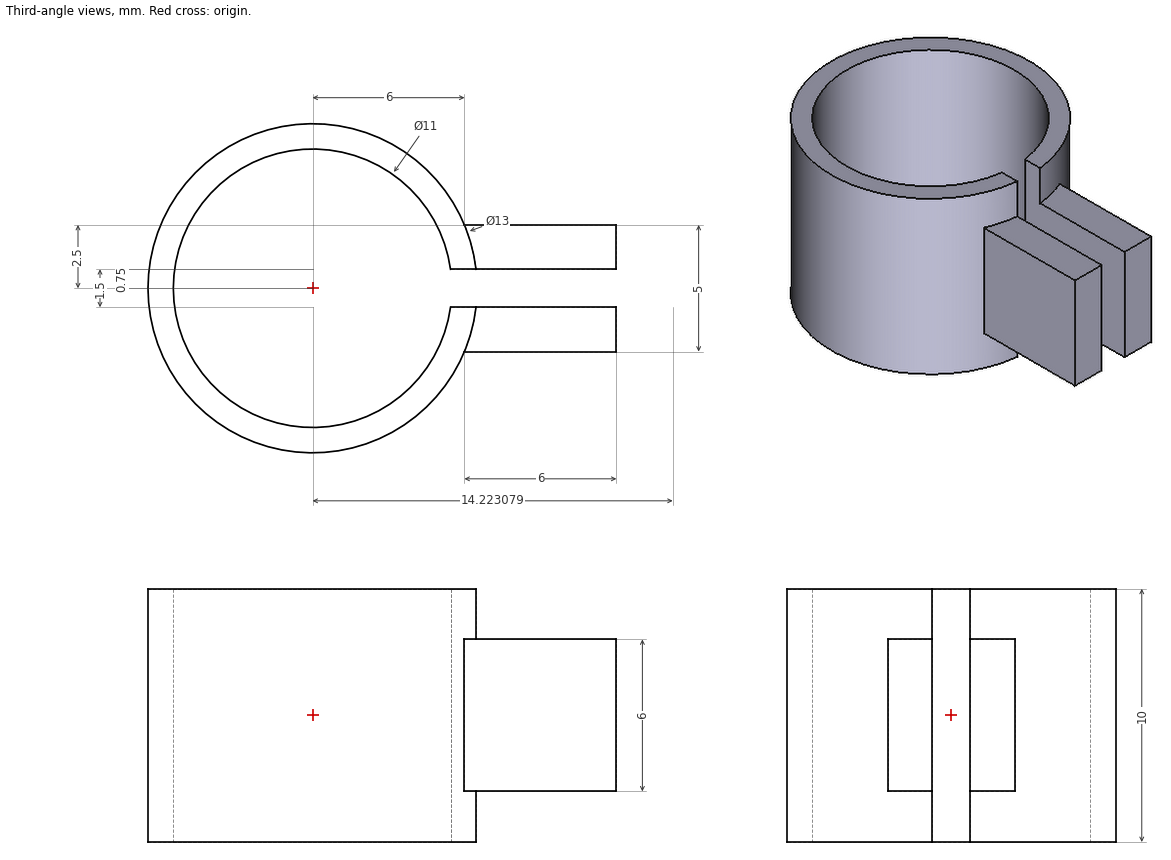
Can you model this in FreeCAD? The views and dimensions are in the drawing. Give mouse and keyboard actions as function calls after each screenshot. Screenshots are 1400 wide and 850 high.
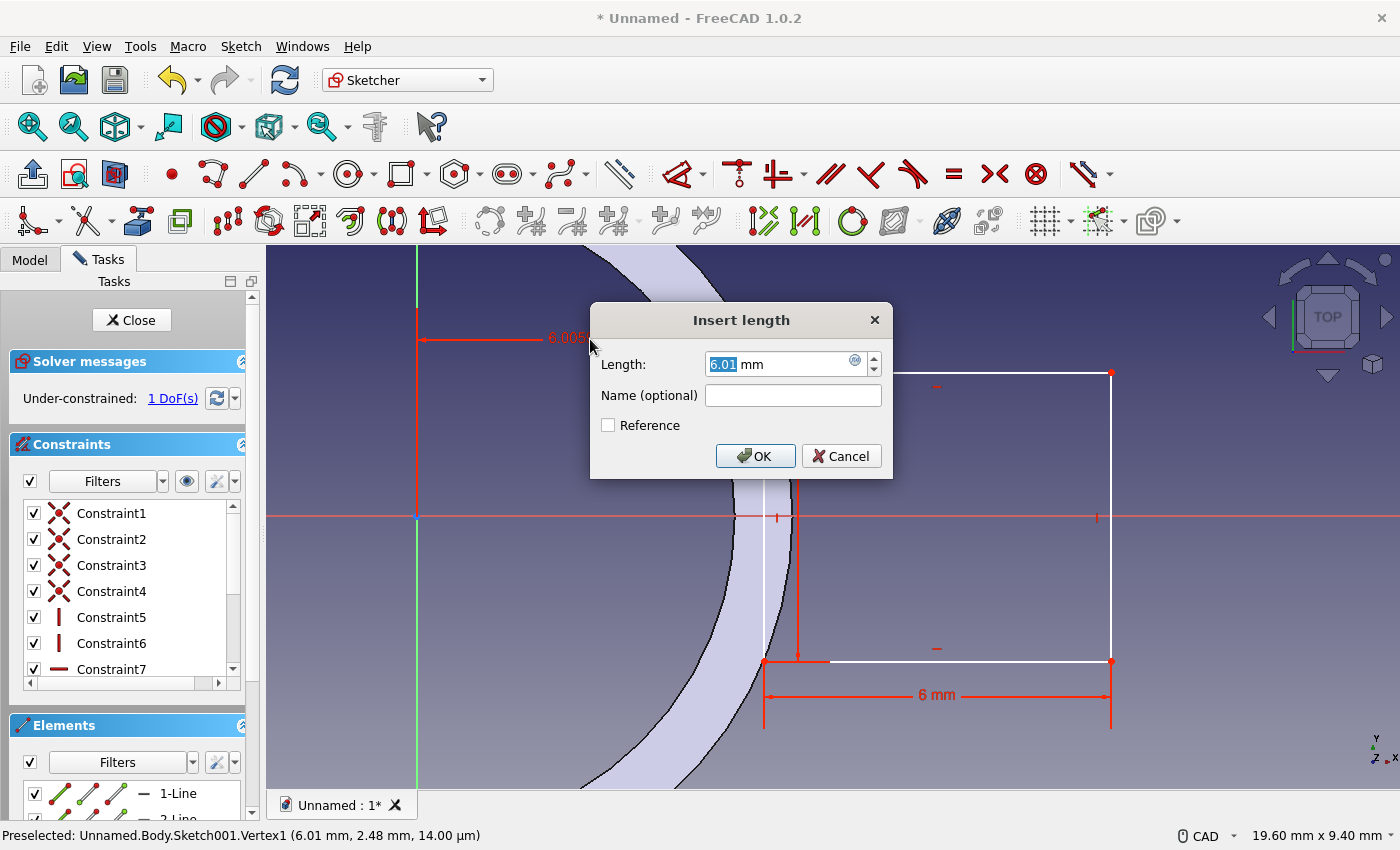
text(6)
key(Return)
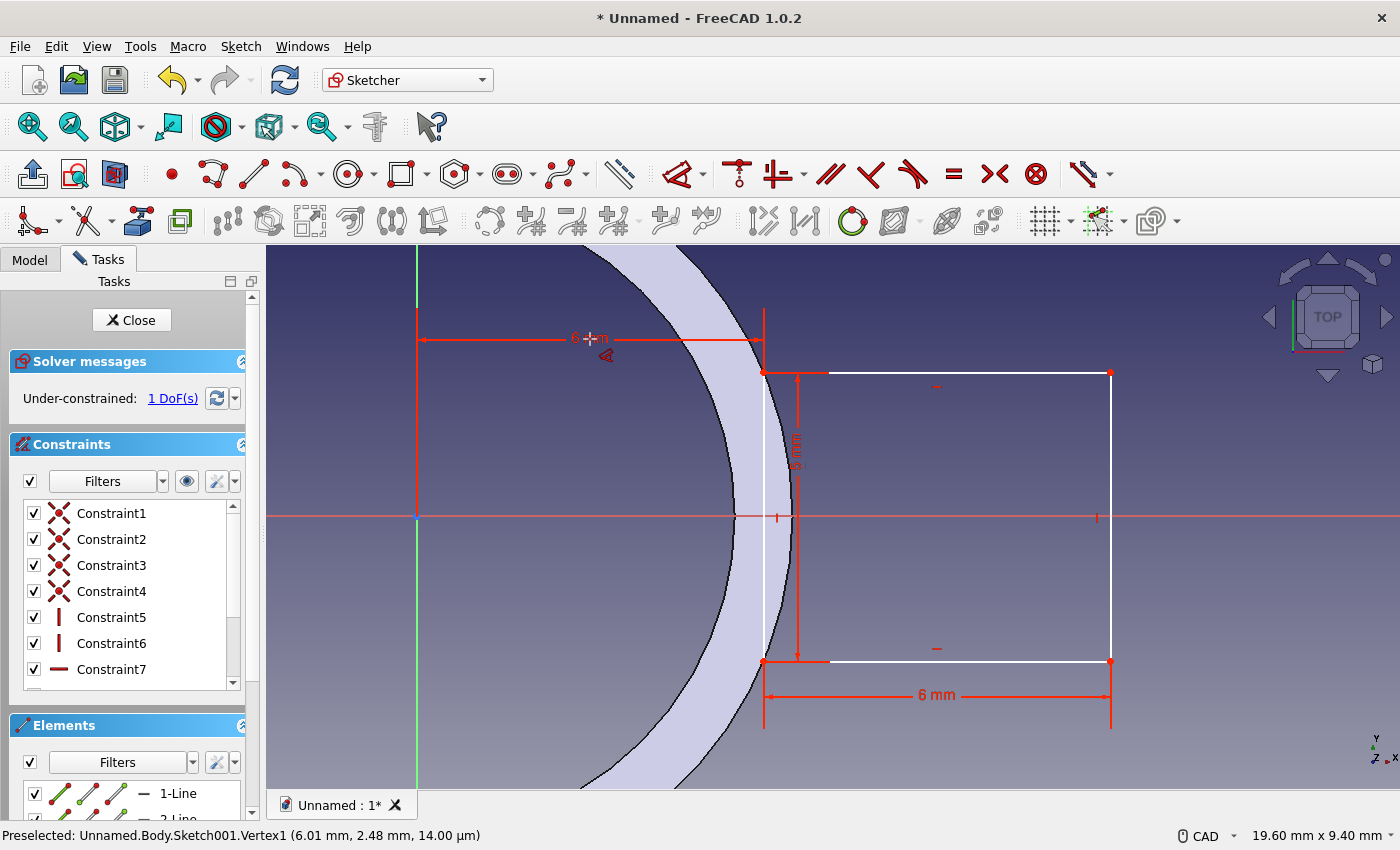
click(764, 373)
click(383, 445)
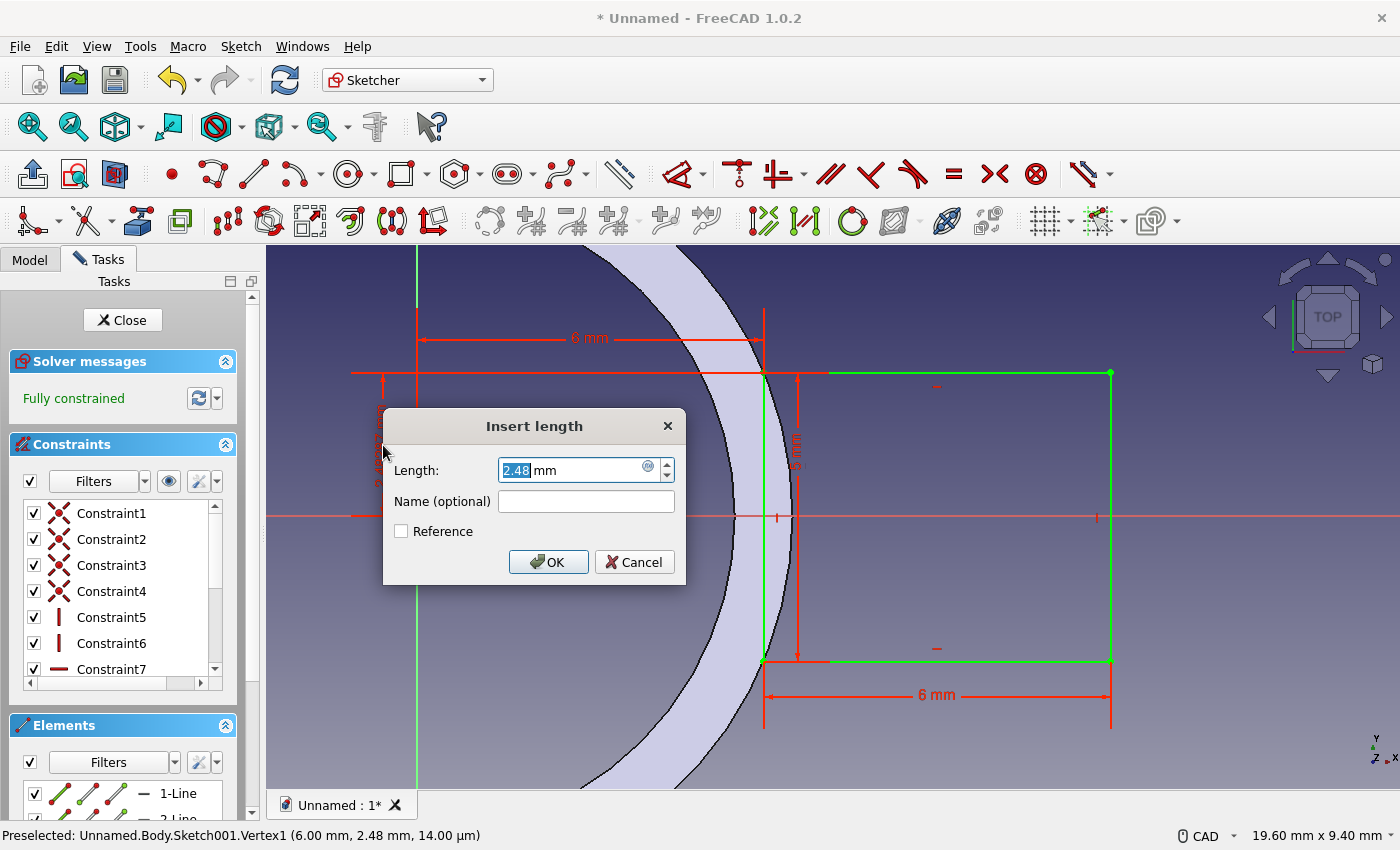
text(2.5)
key(Return)
key(Escape)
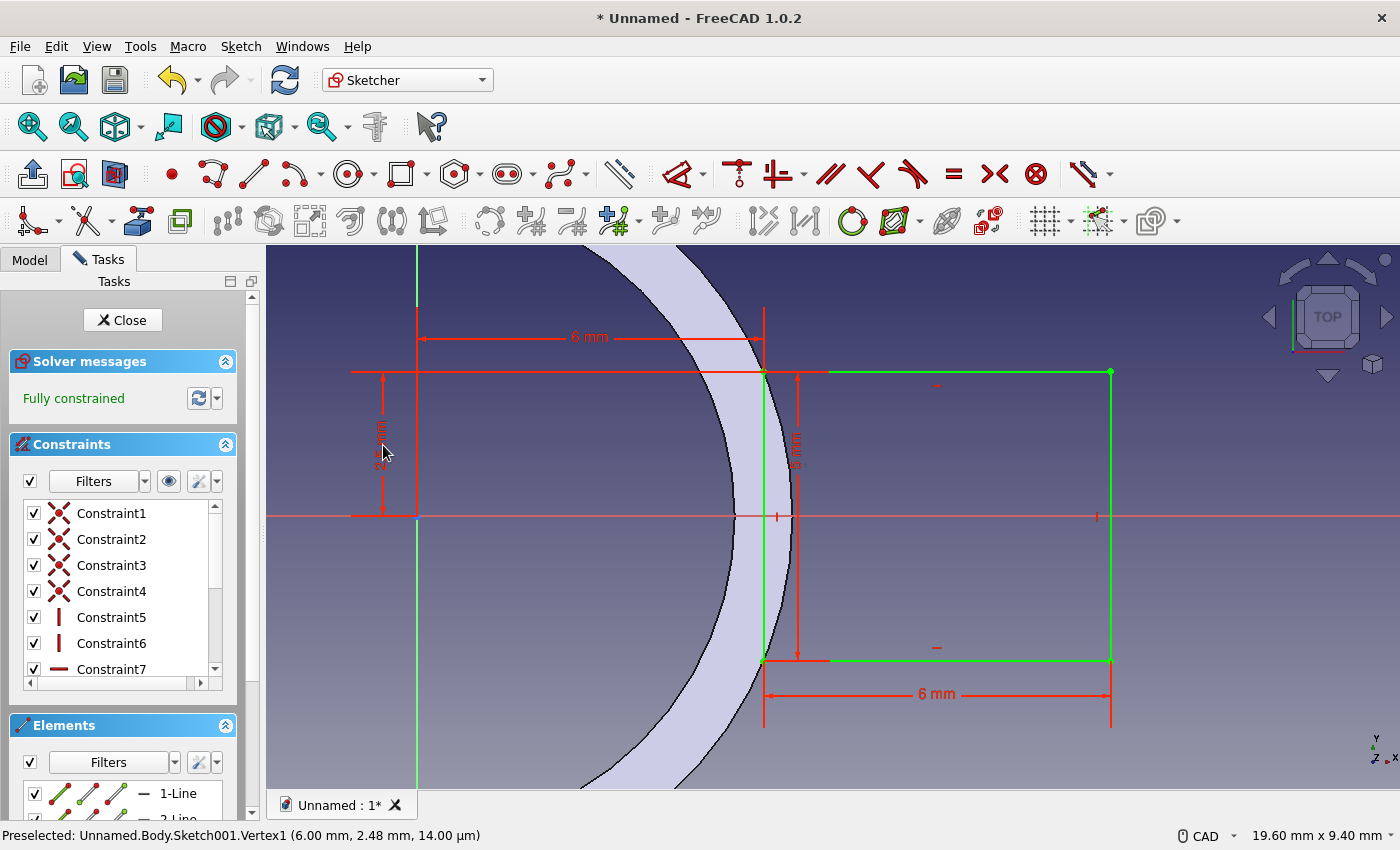
click(123, 320)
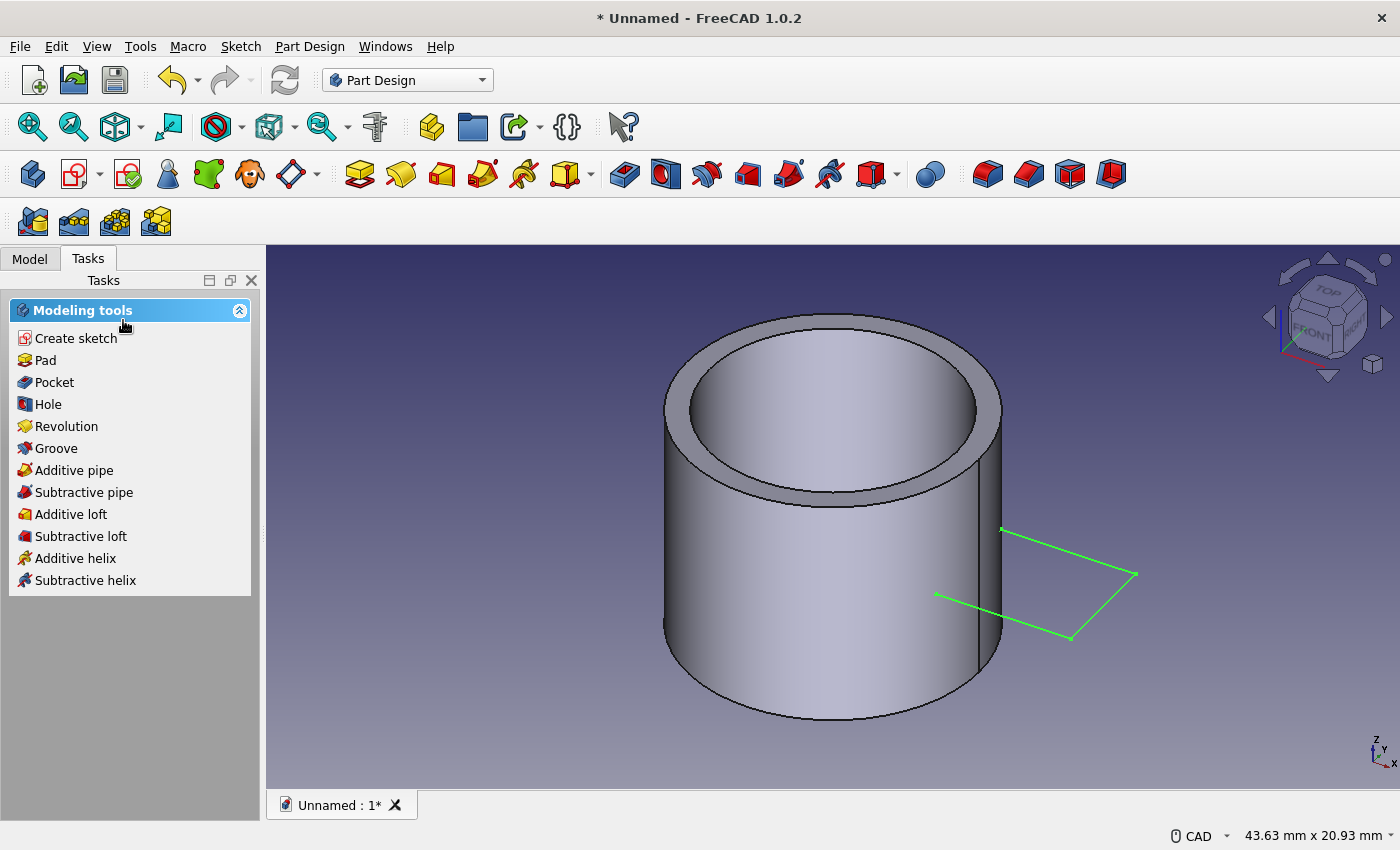
click(360, 174)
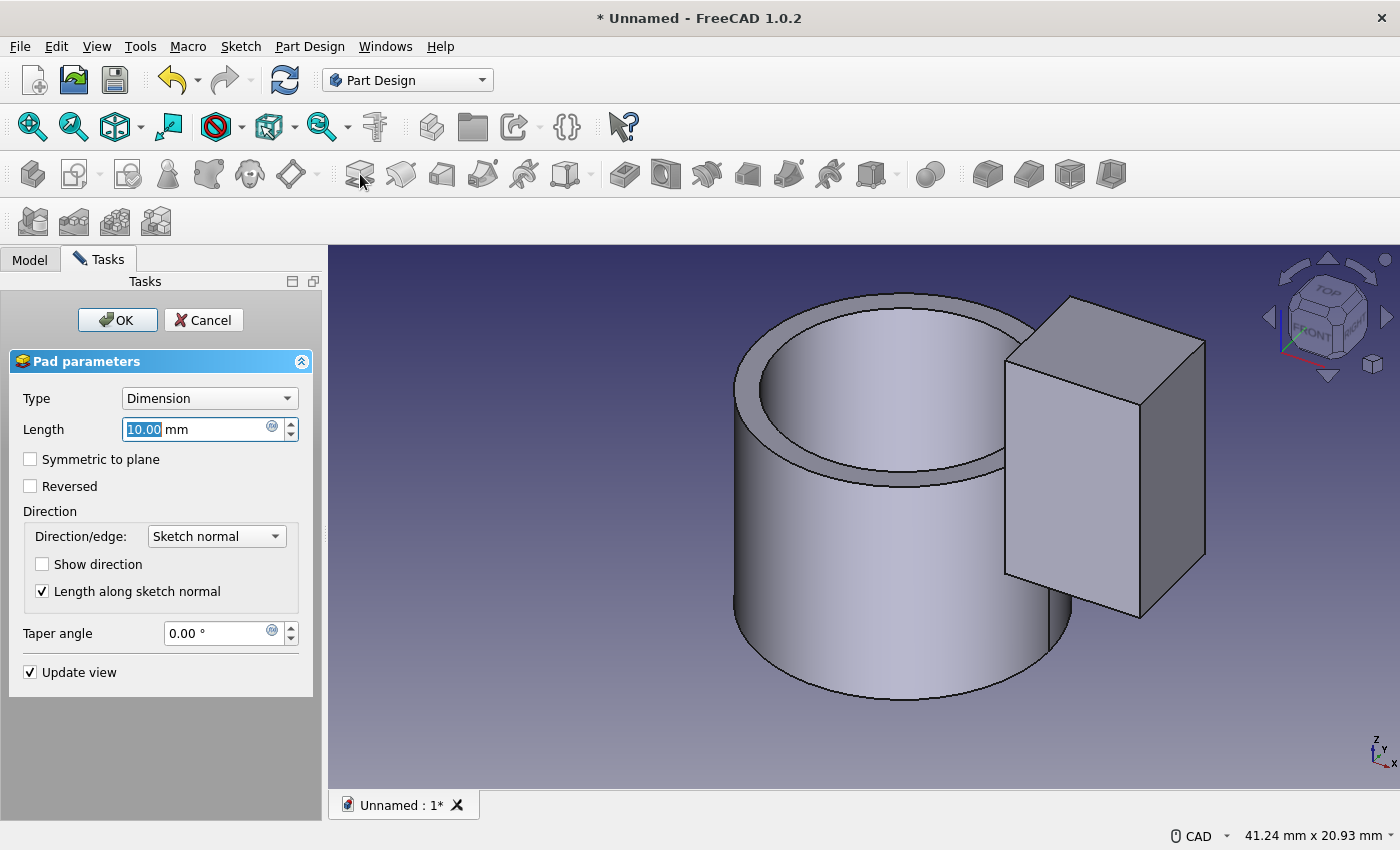
text(6)
key(Tab)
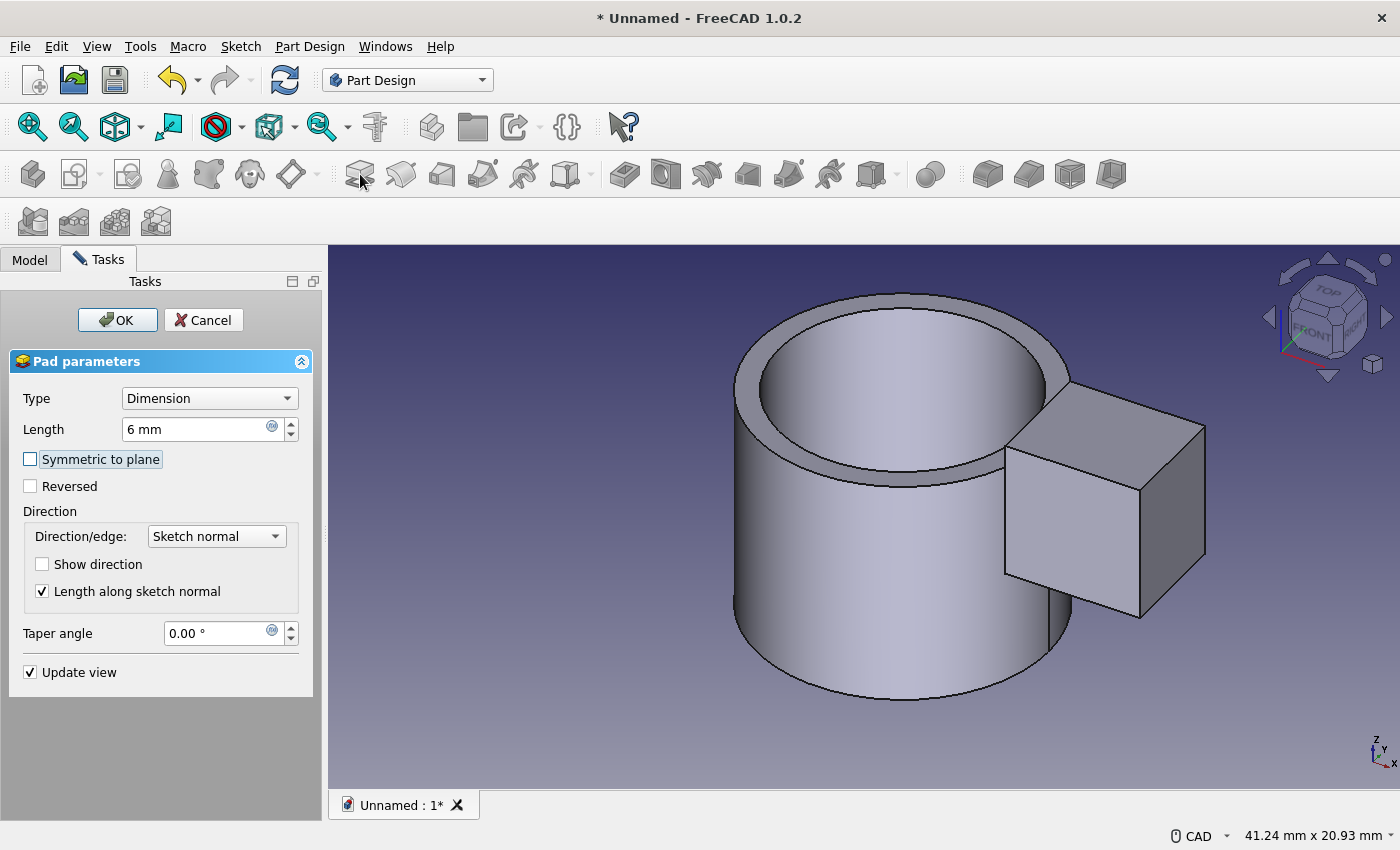
click(31, 459)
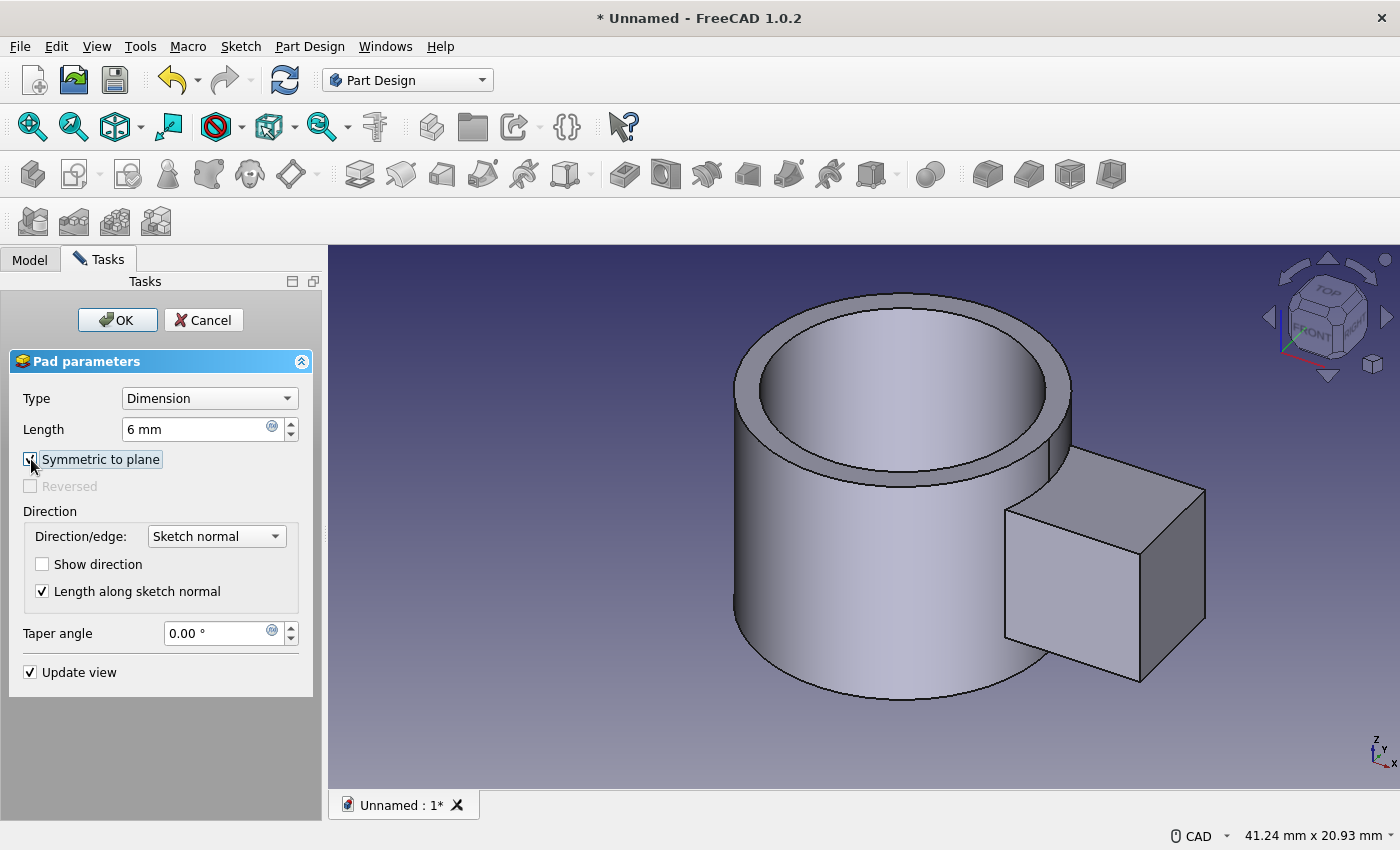
click(118, 320)